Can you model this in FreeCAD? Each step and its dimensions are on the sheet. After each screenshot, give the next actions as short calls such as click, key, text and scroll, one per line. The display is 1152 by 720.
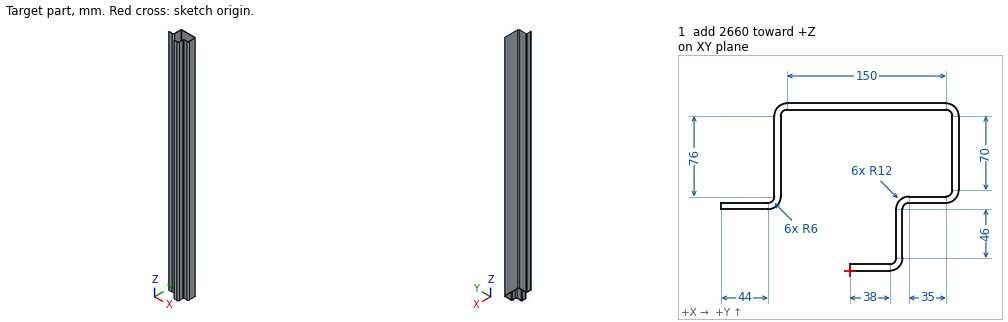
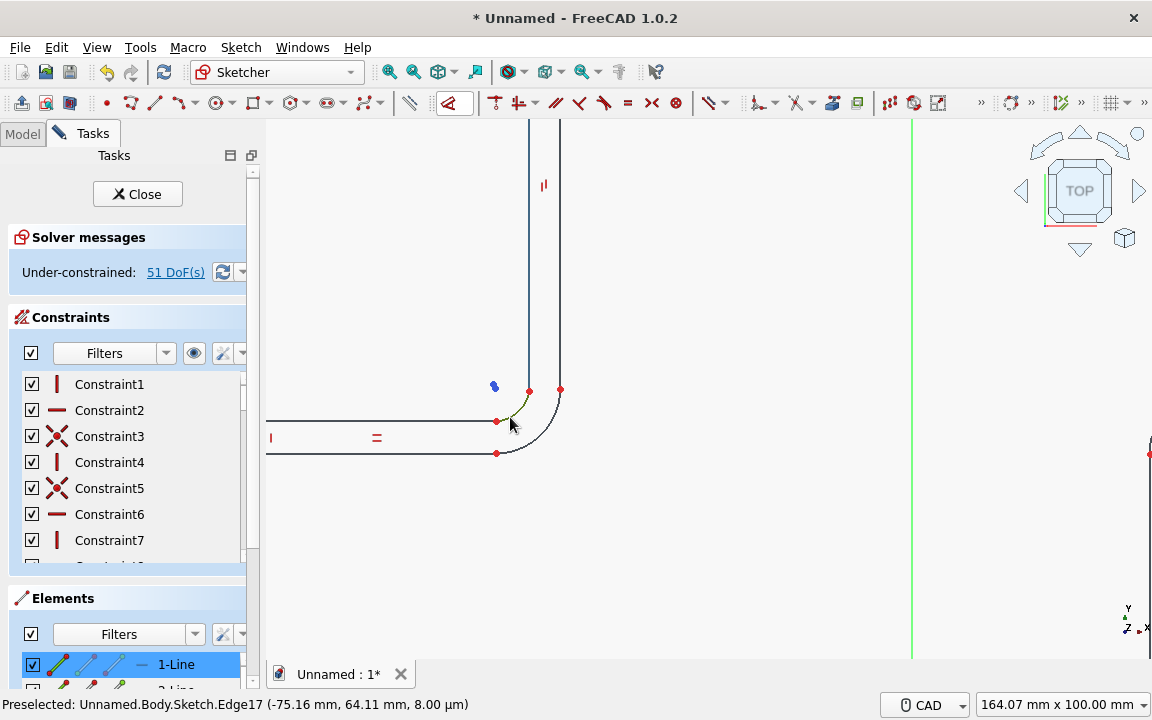
key(t)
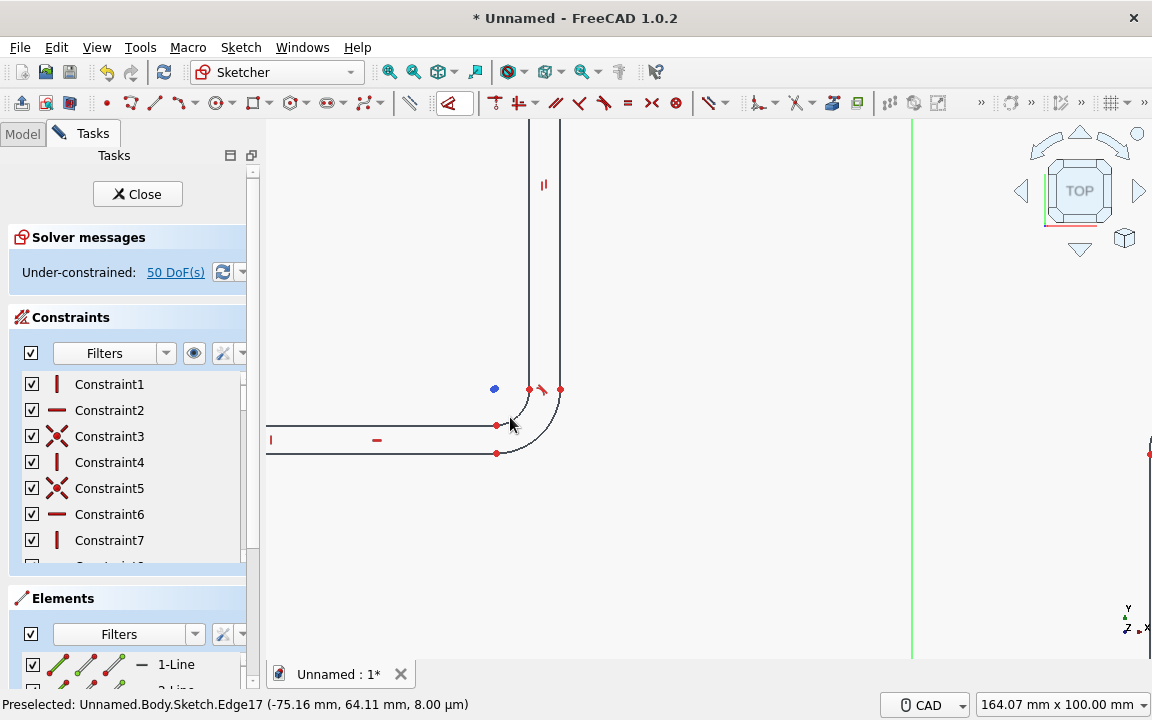
click(529, 267)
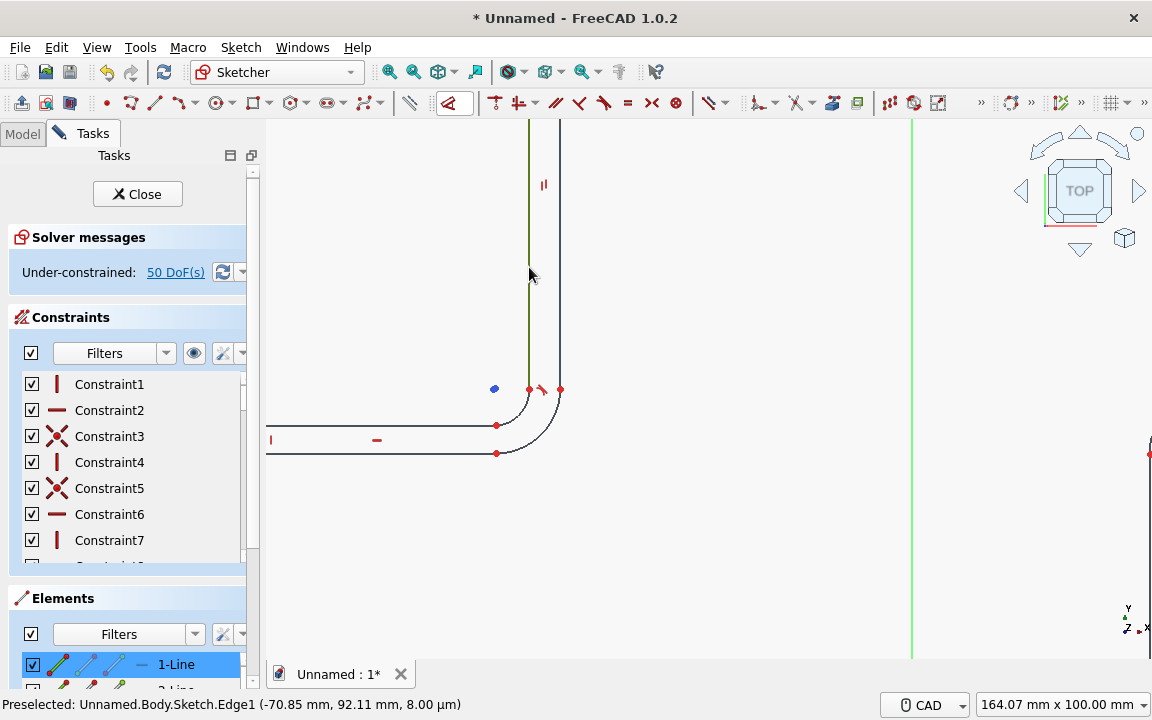
scroll(511, 418, down, 5)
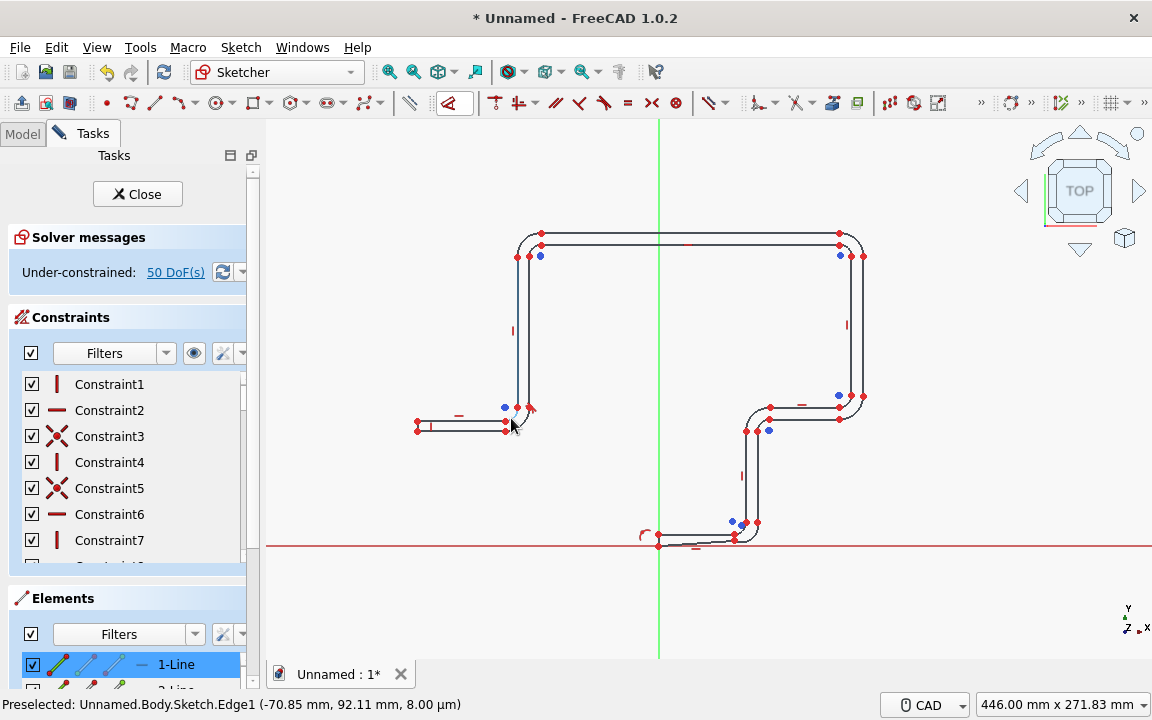
click(530, 236)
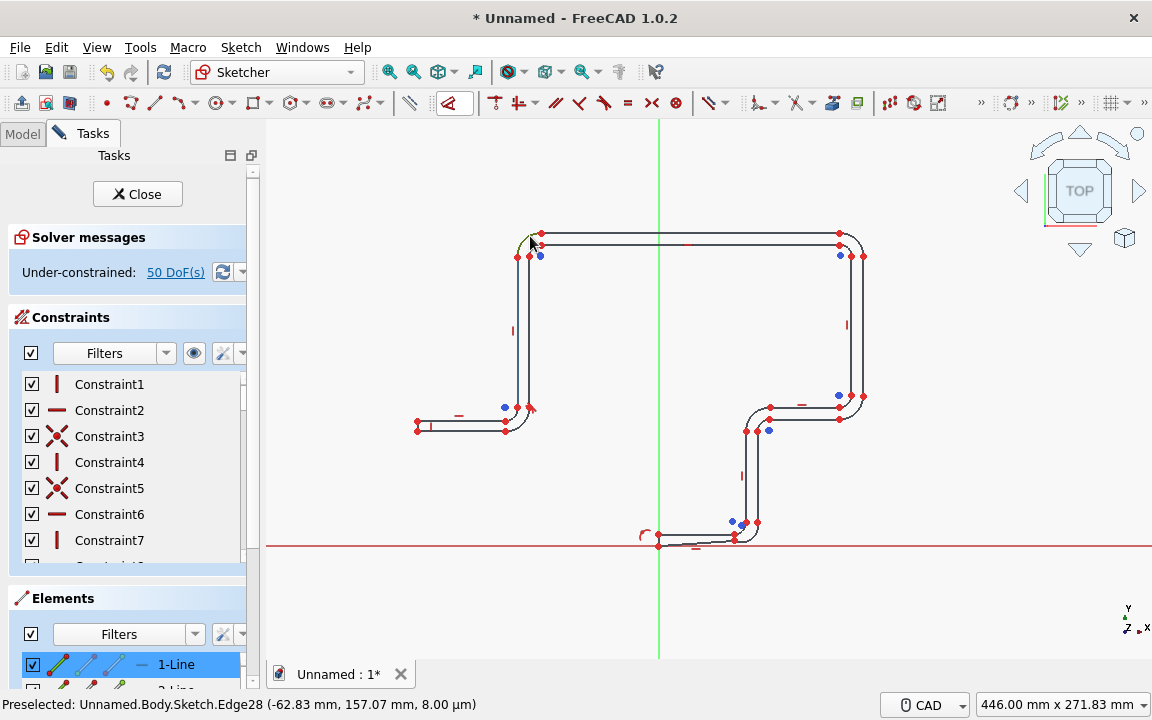
click(604, 104)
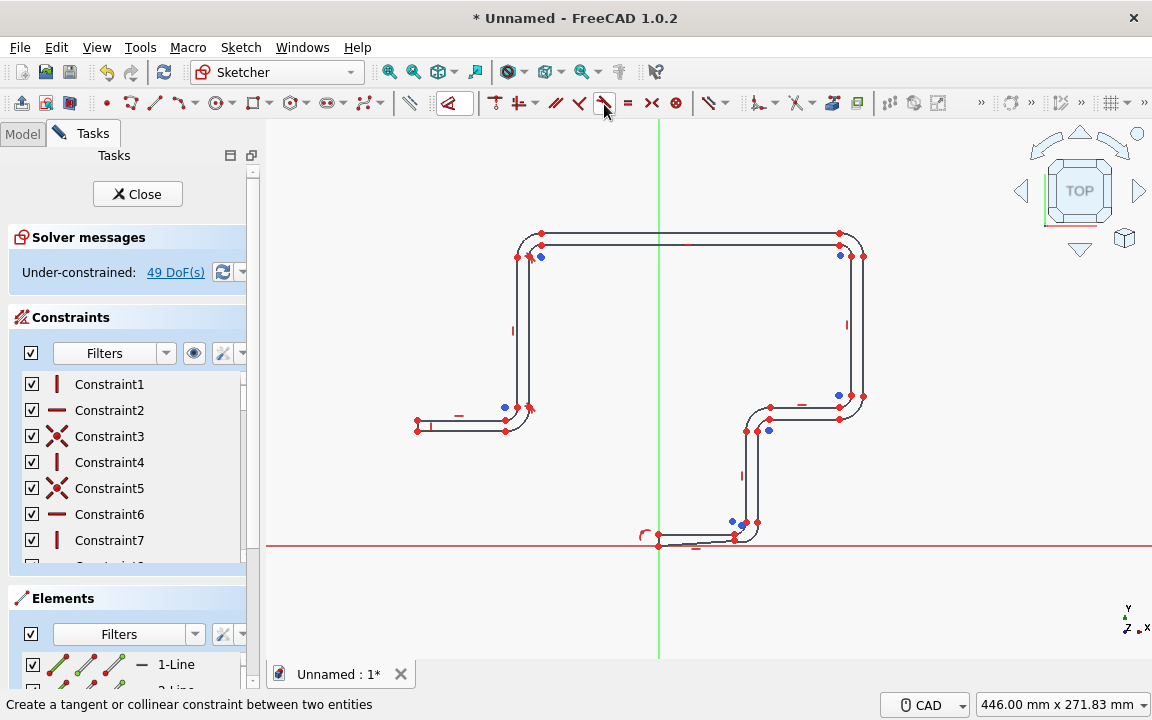
scroll(480, 421, up, 2)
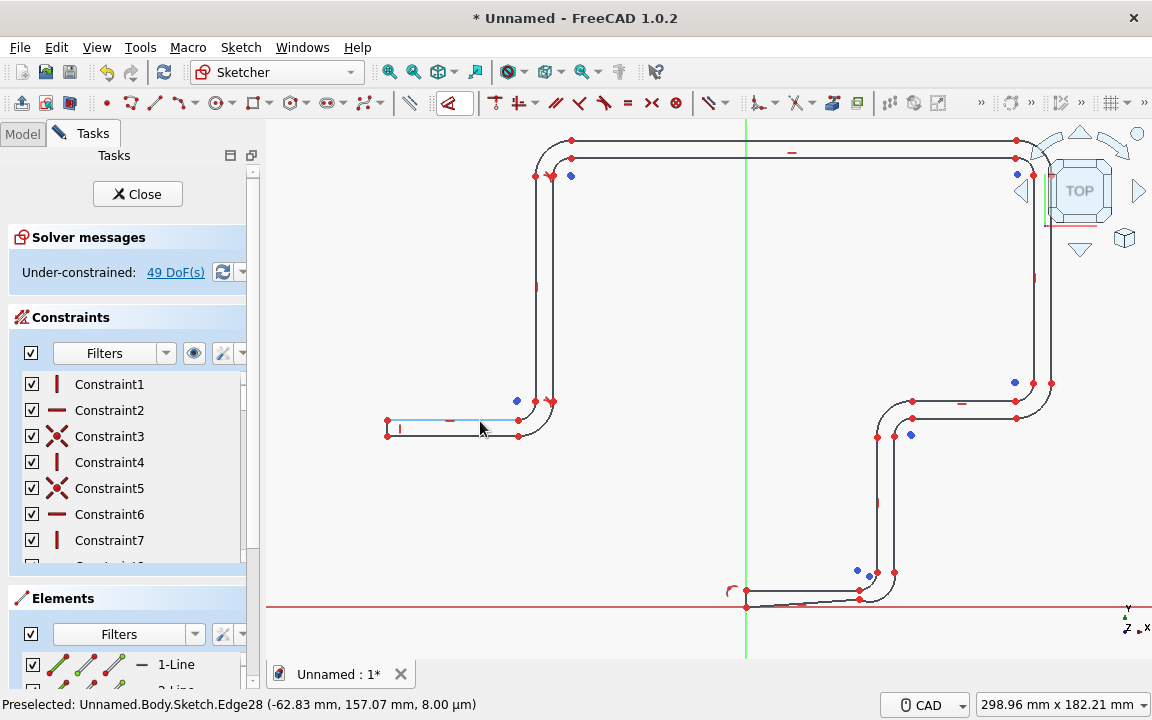
click(479, 420)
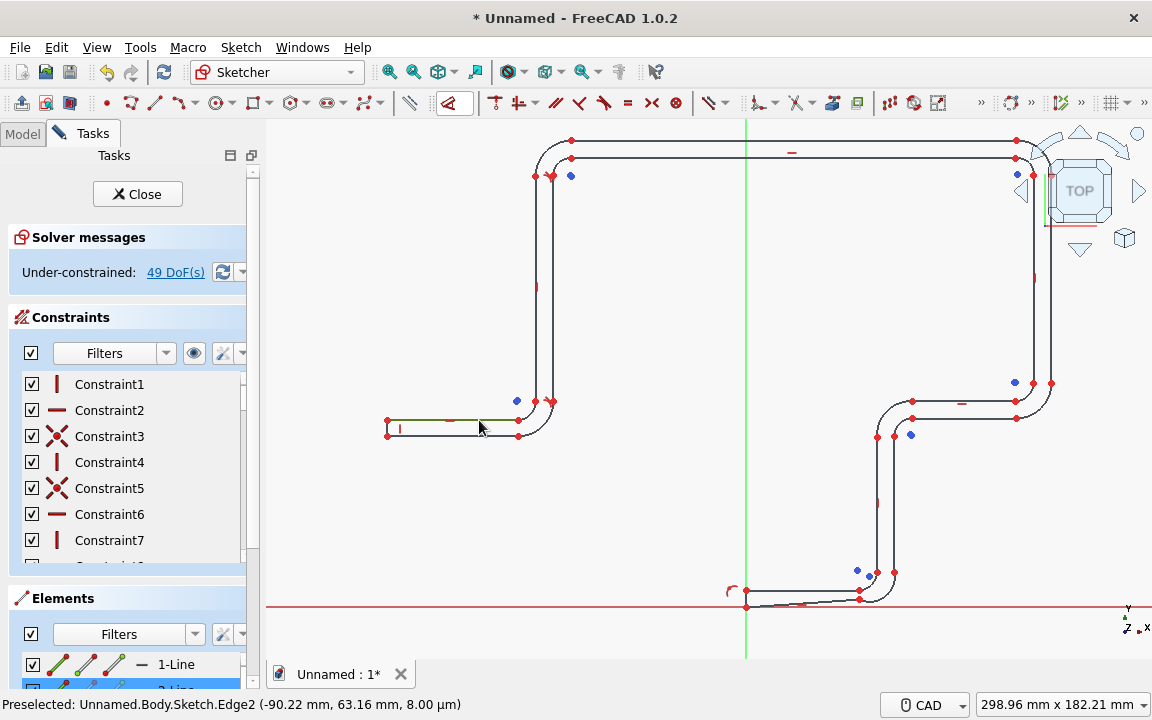
click(531, 414)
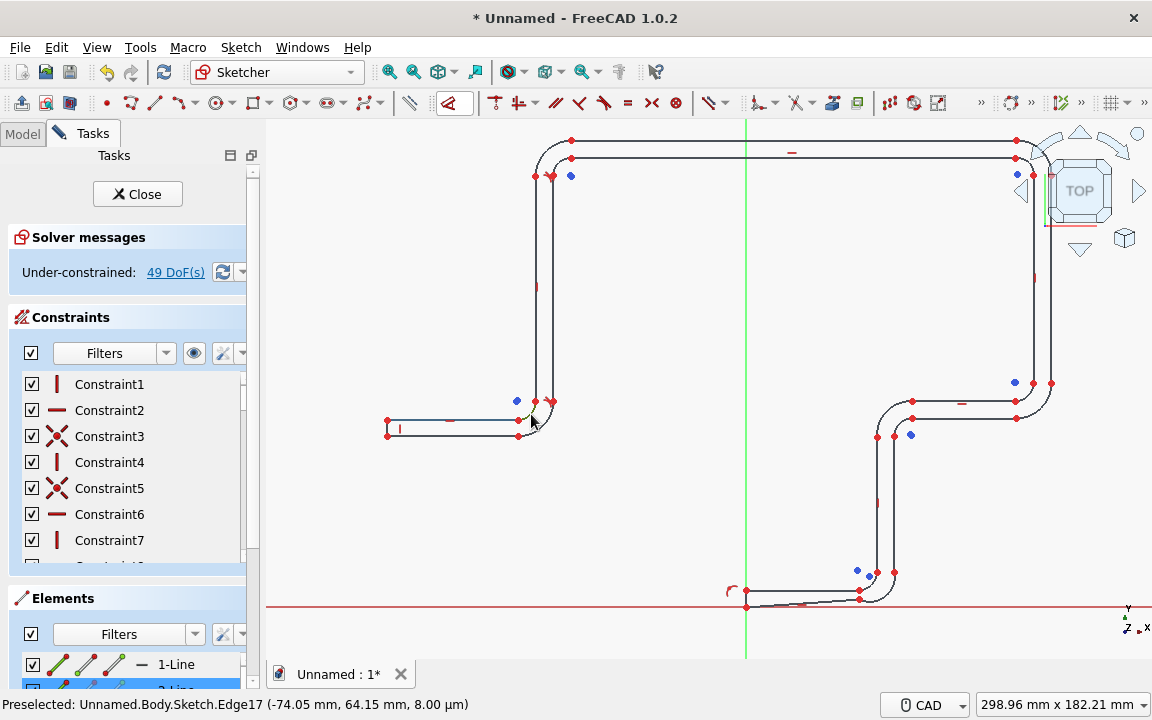
key(t)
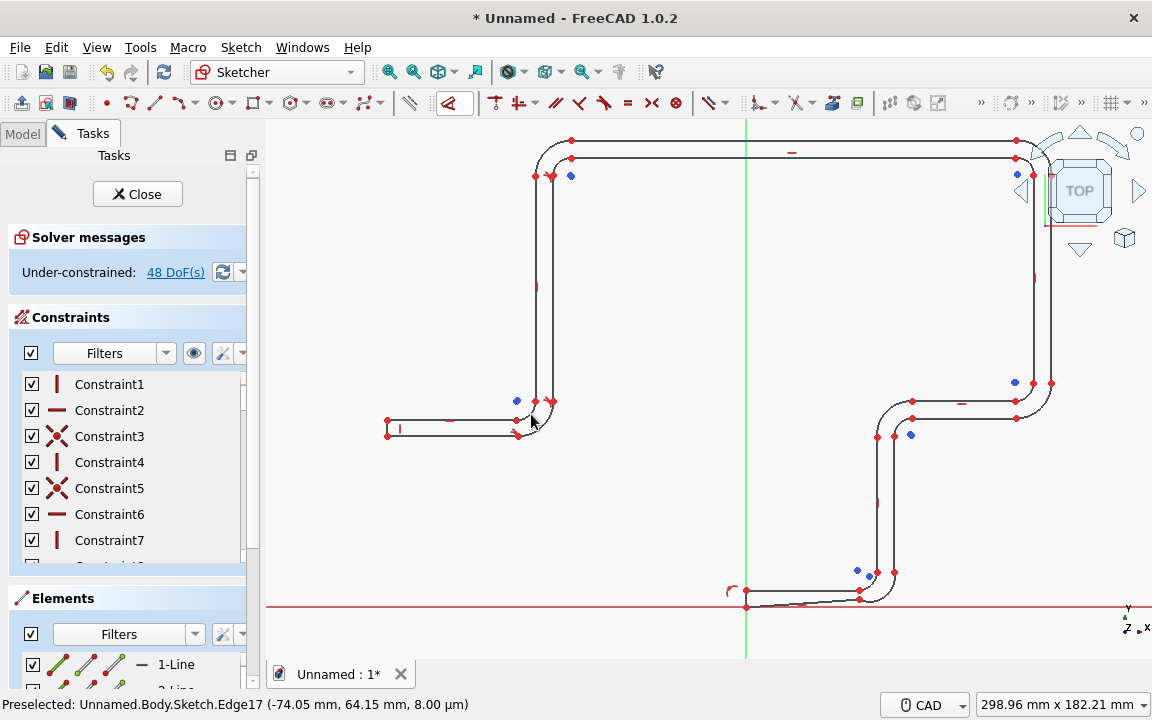
click(427, 436)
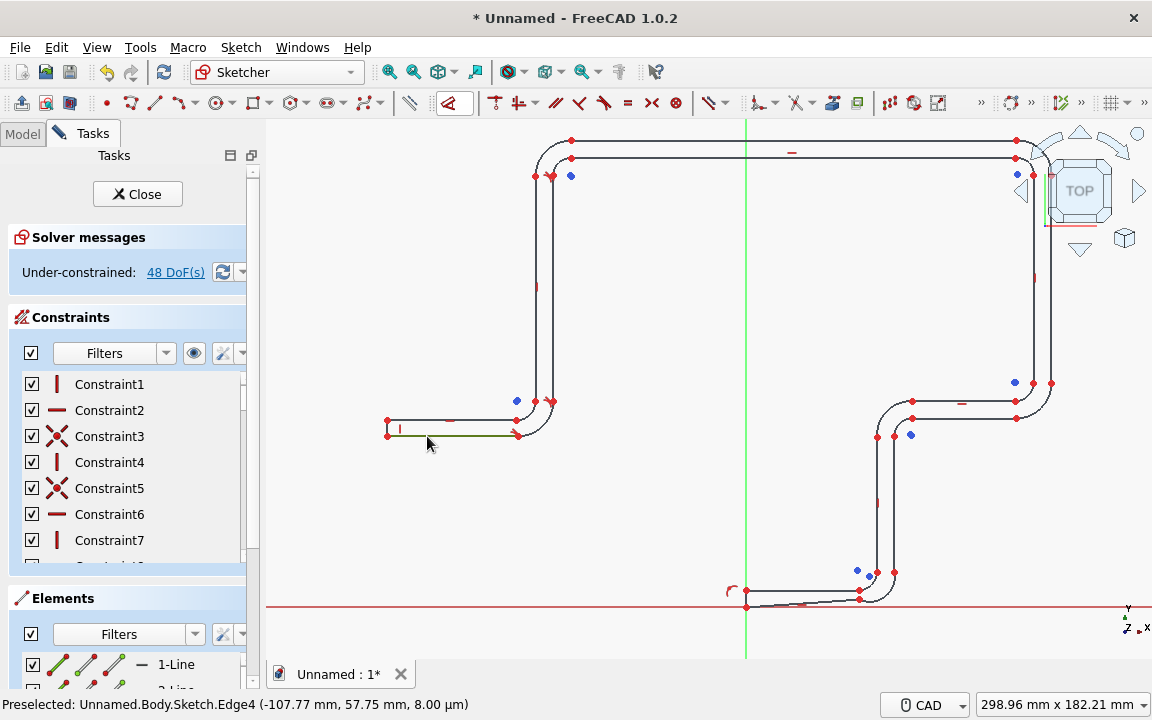
click(534, 432)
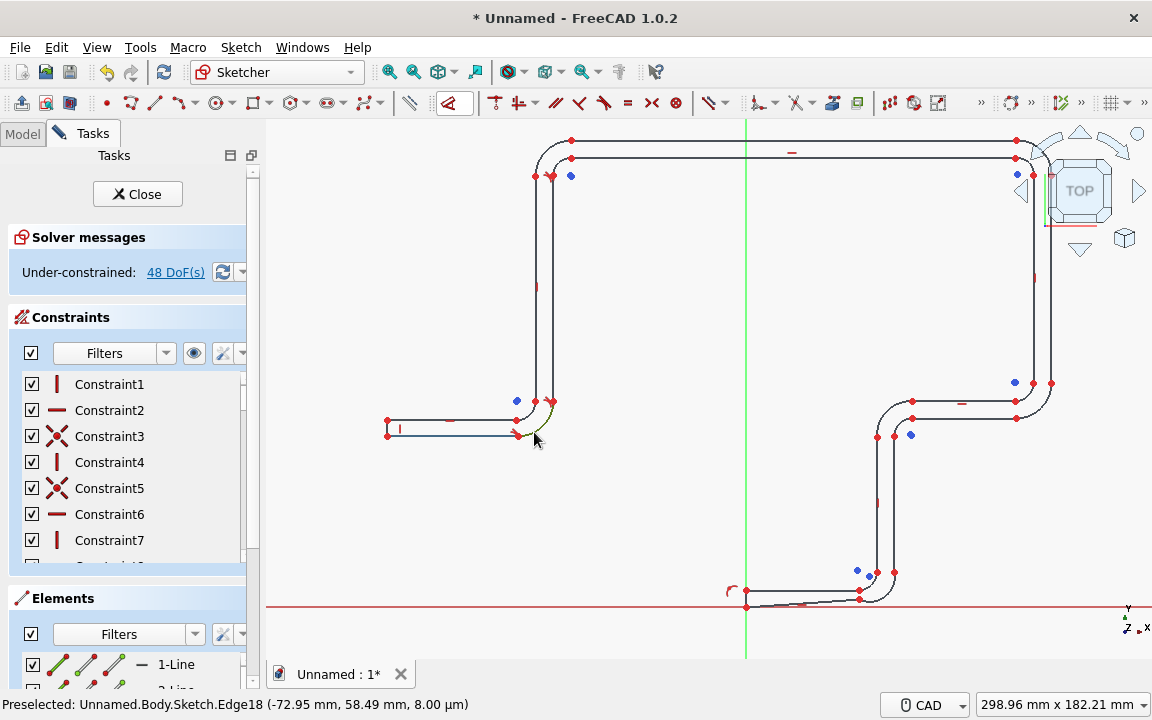
key(t)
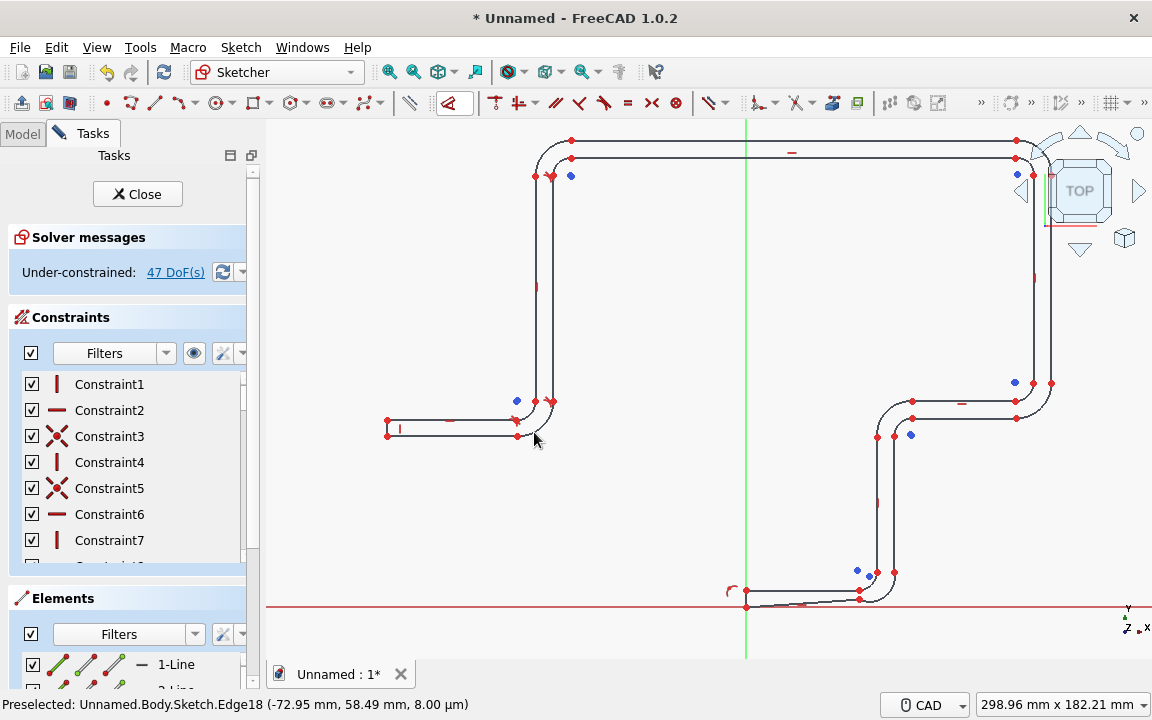
click(553, 333)